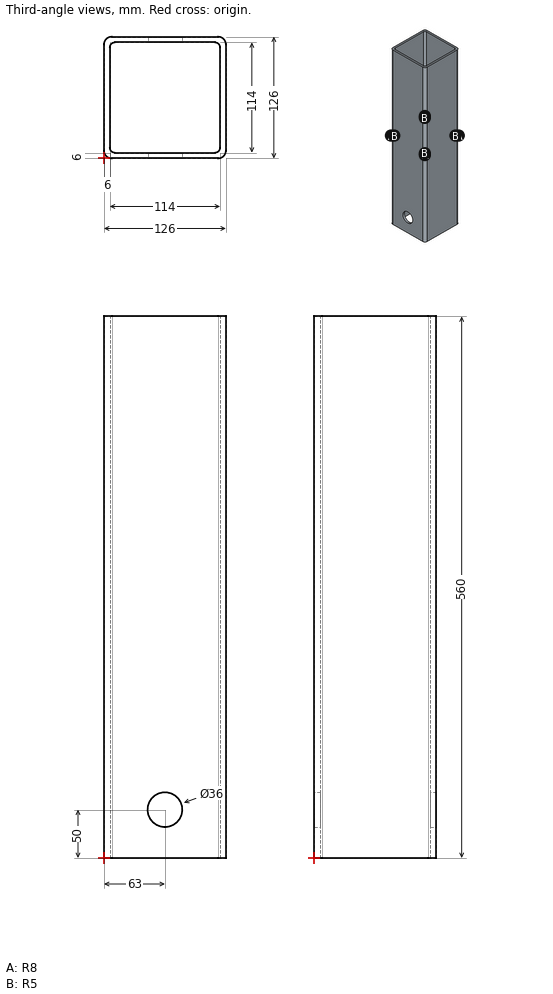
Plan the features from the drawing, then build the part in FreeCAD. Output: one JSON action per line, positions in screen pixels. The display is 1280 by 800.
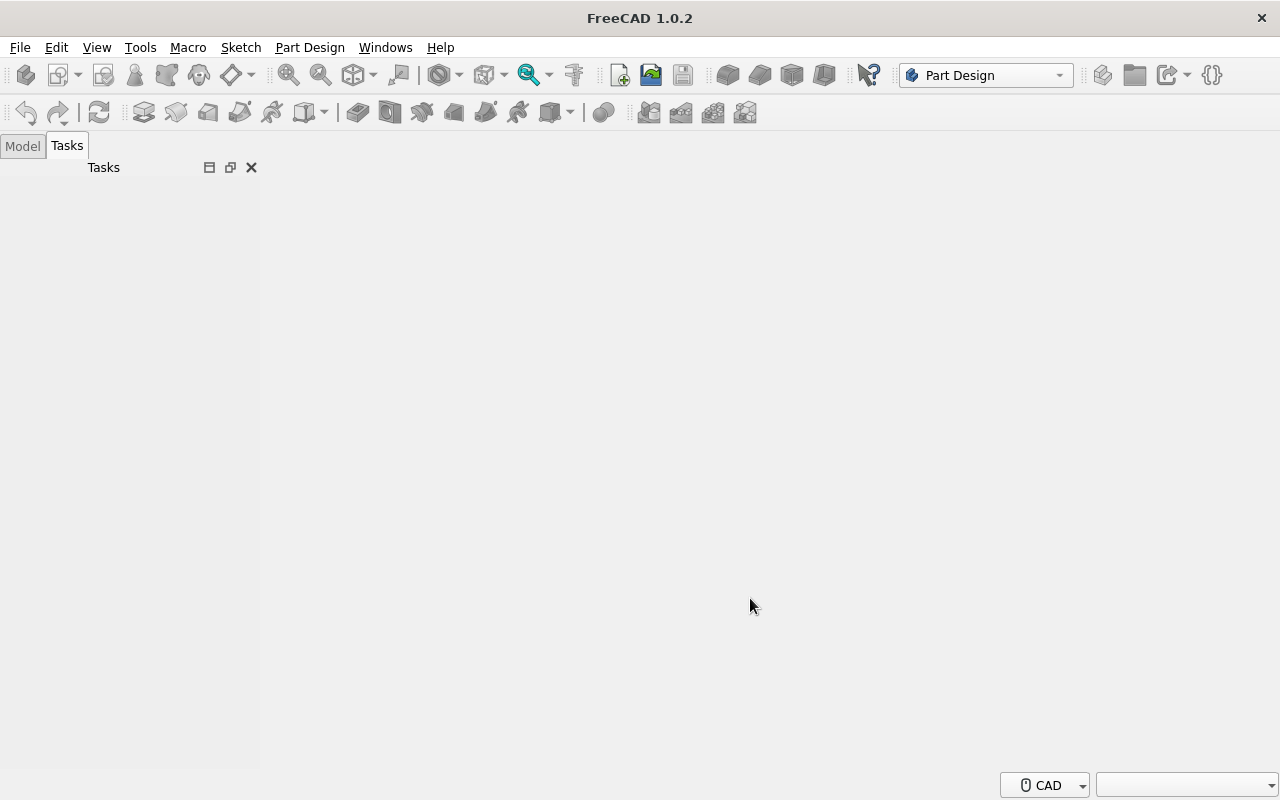
{"action": "left_click", "coordinate": [620, 76]}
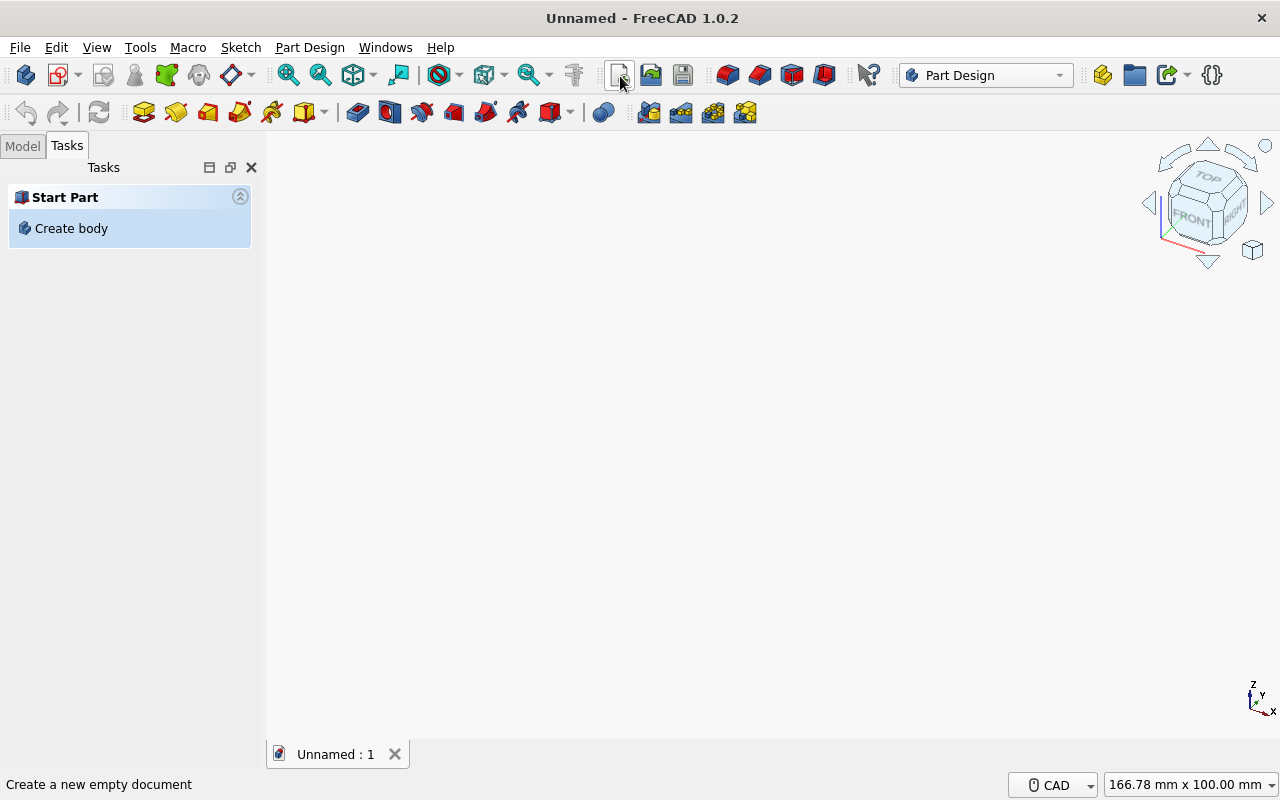
{"action": "left_click", "coordinate": [58, 76]}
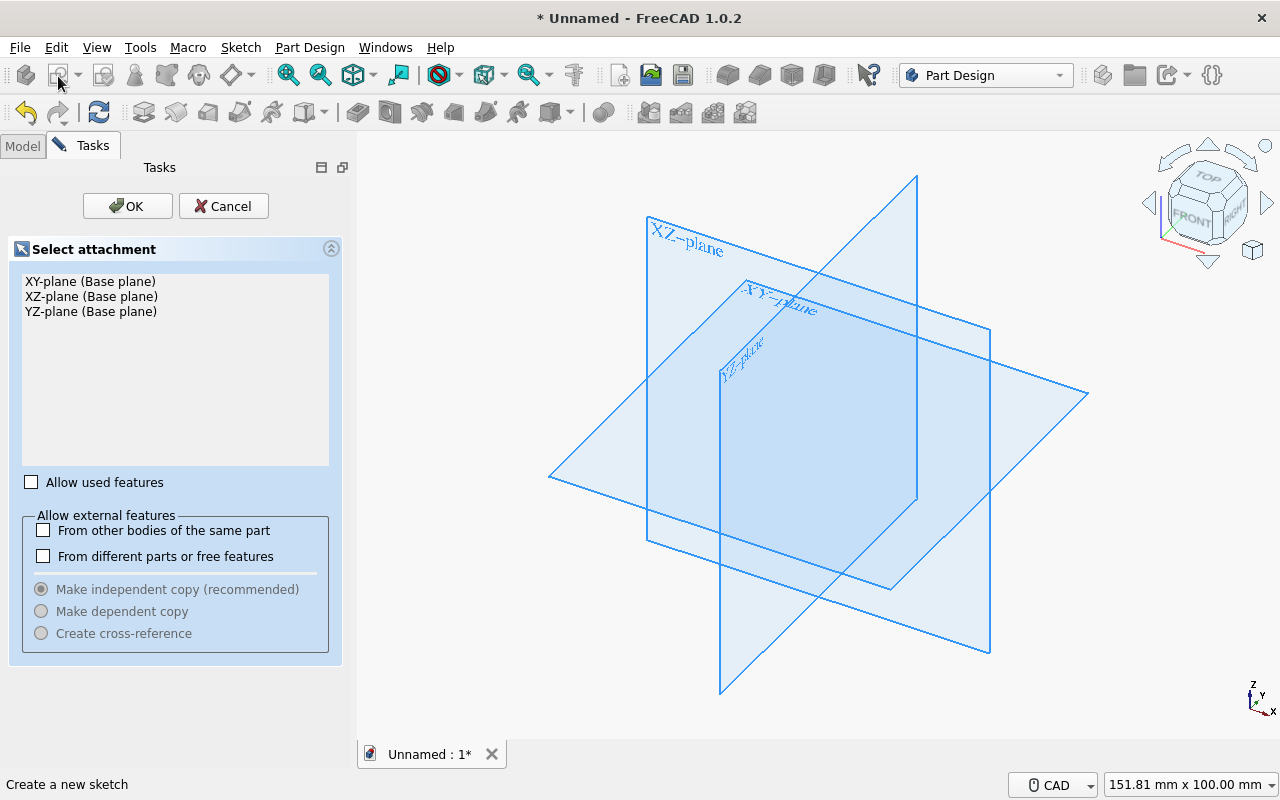
{"action": "left_click", "coordinate": [82, 282]}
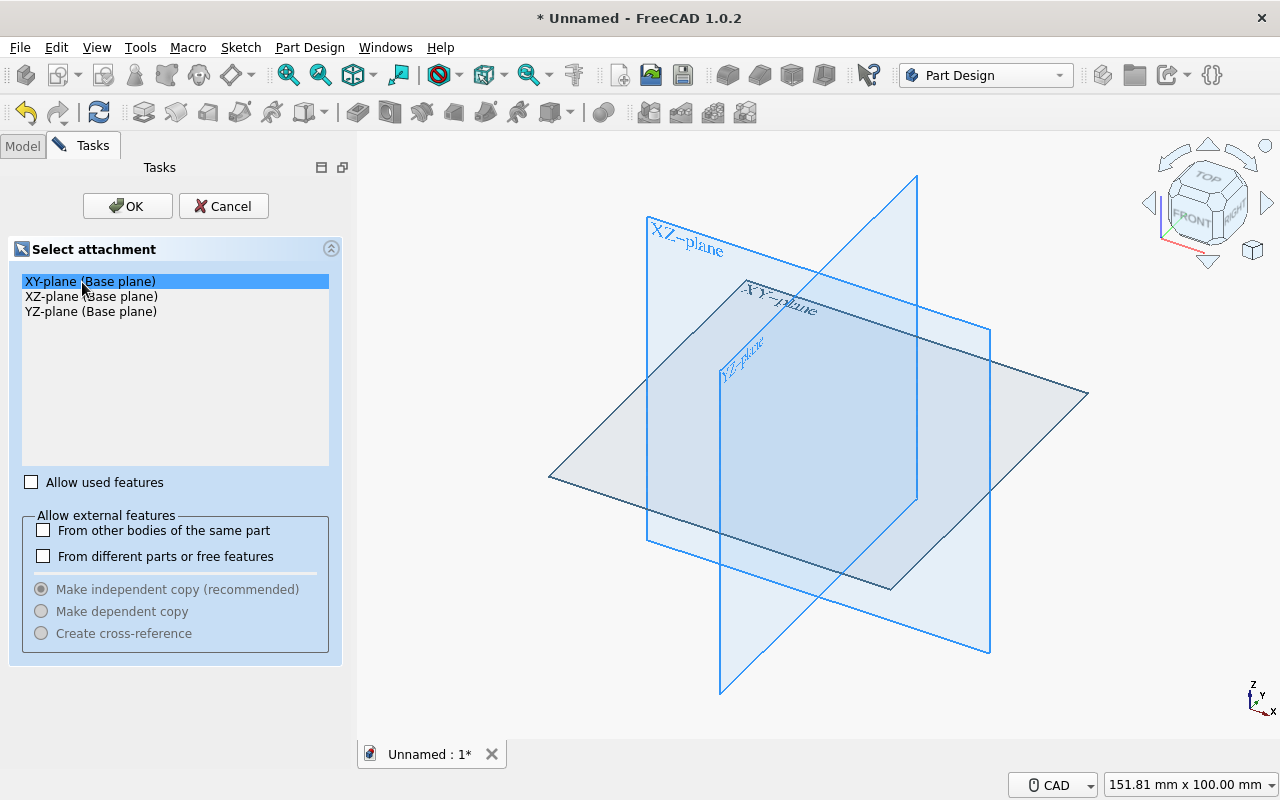
{"action": "left_click", "coordinate": [128, 206]}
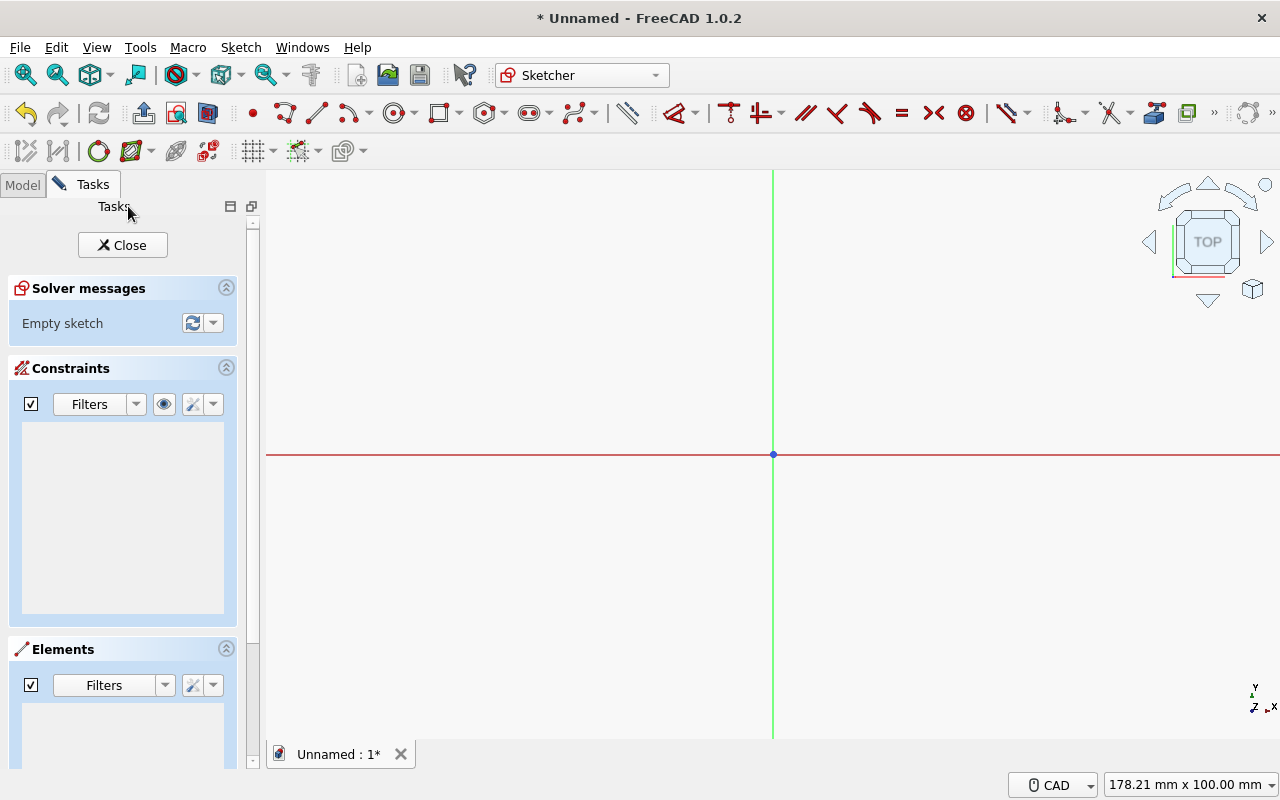
{"action": "scroll", "coordinate": [356, 711], "scroll_direction": "down", "scroll_amount": 4}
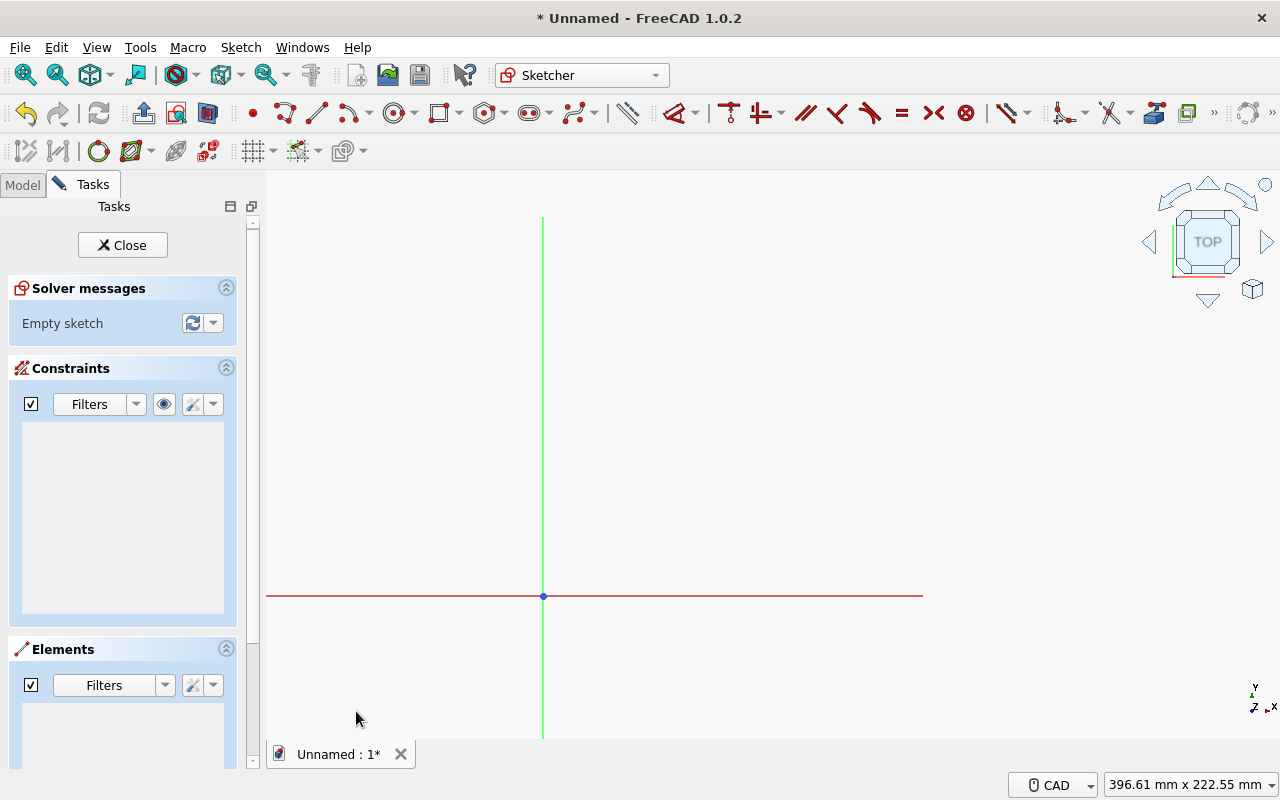
{"action": "left_click", "coordinate": [440, 114]}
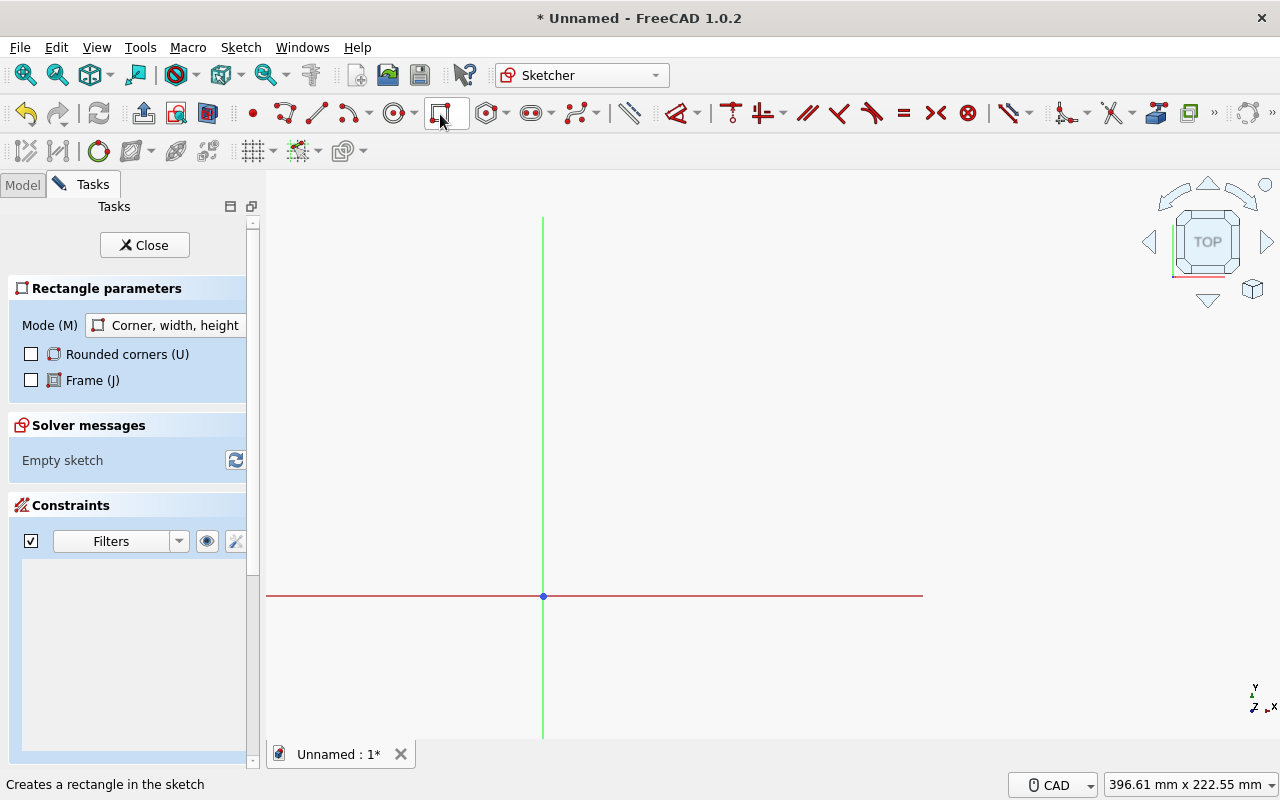
{"action": "left_click", "coordinate": [543, 596]}
{"action": "mouse_move", "coordinate": [866, 274]}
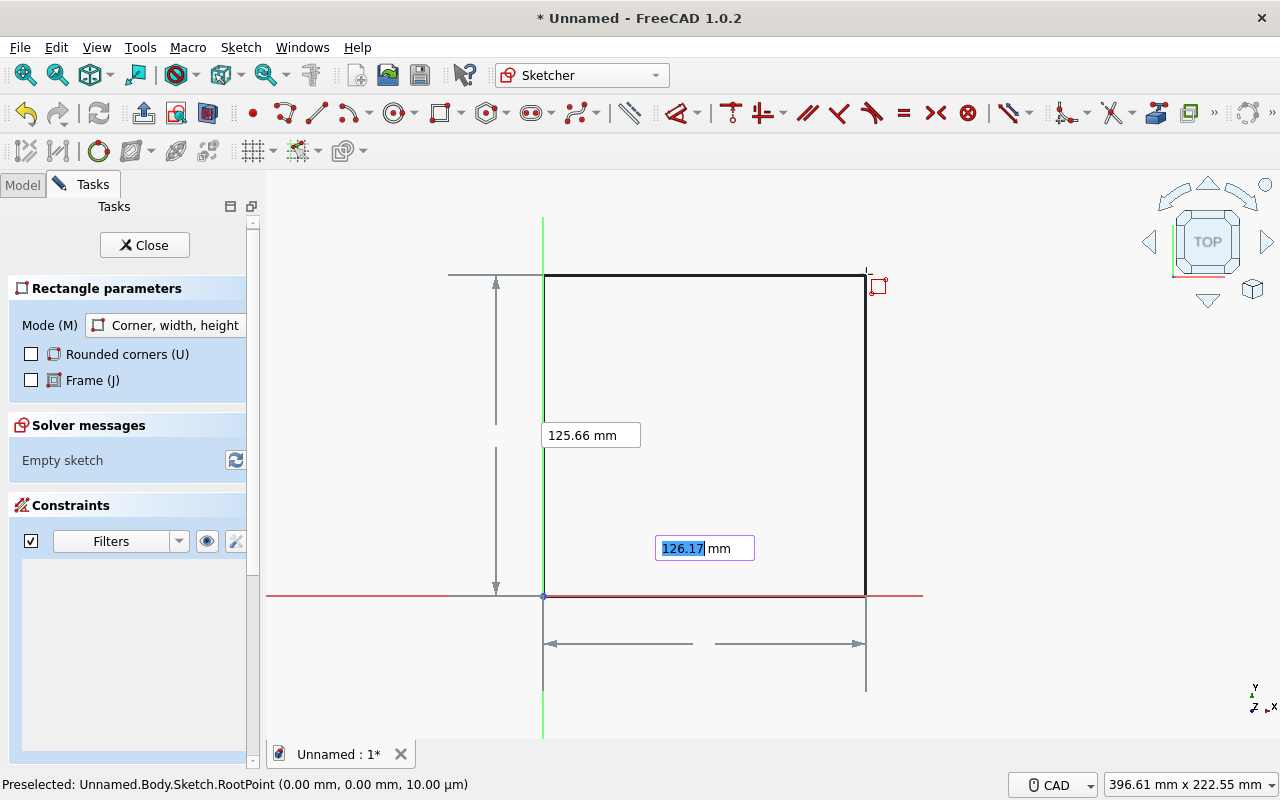
{"action": "type", "text": "126"}
{"action": "key", "text": "Tab"}
{"action": "type", "text": "126"}
{"action": "key", "text": "Return"}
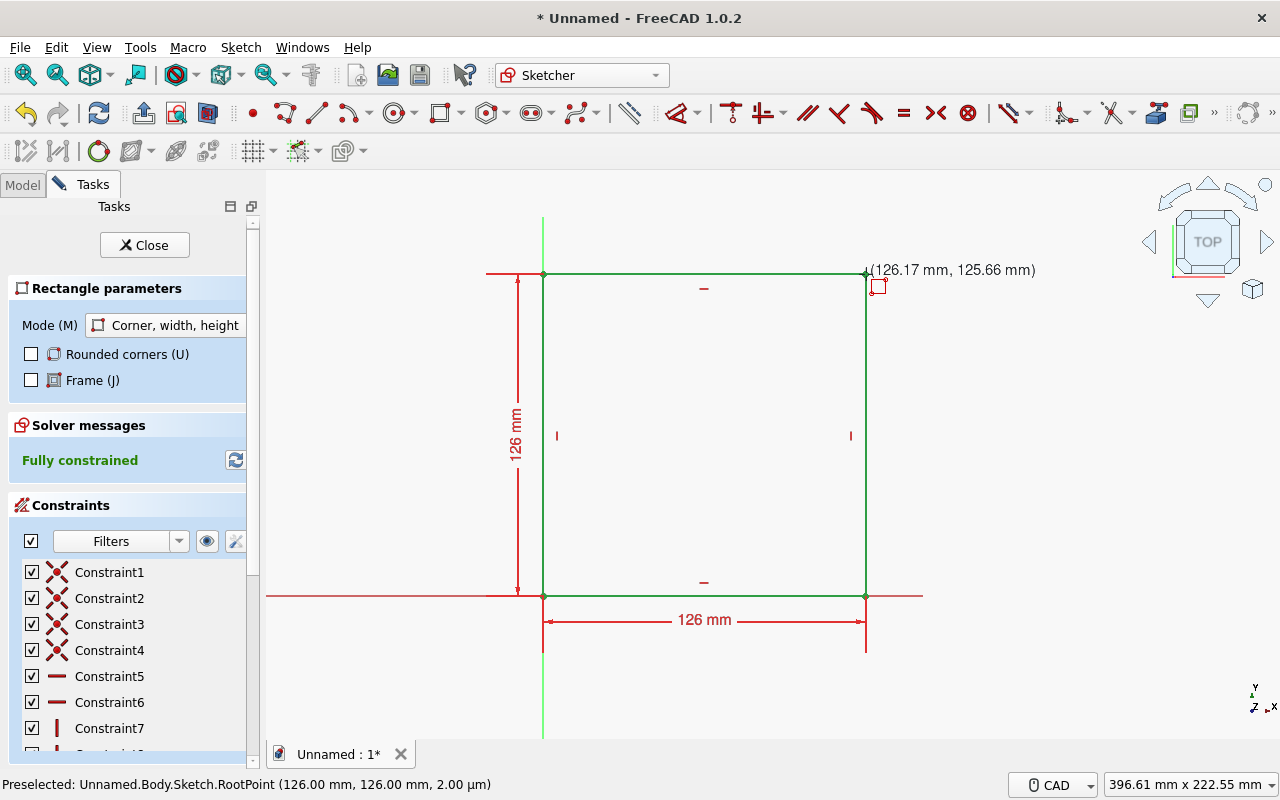
{"action": "left_click", "coordinate": [559, 289]}
{"action": "mouse_move", "coordinate": [850, 581]}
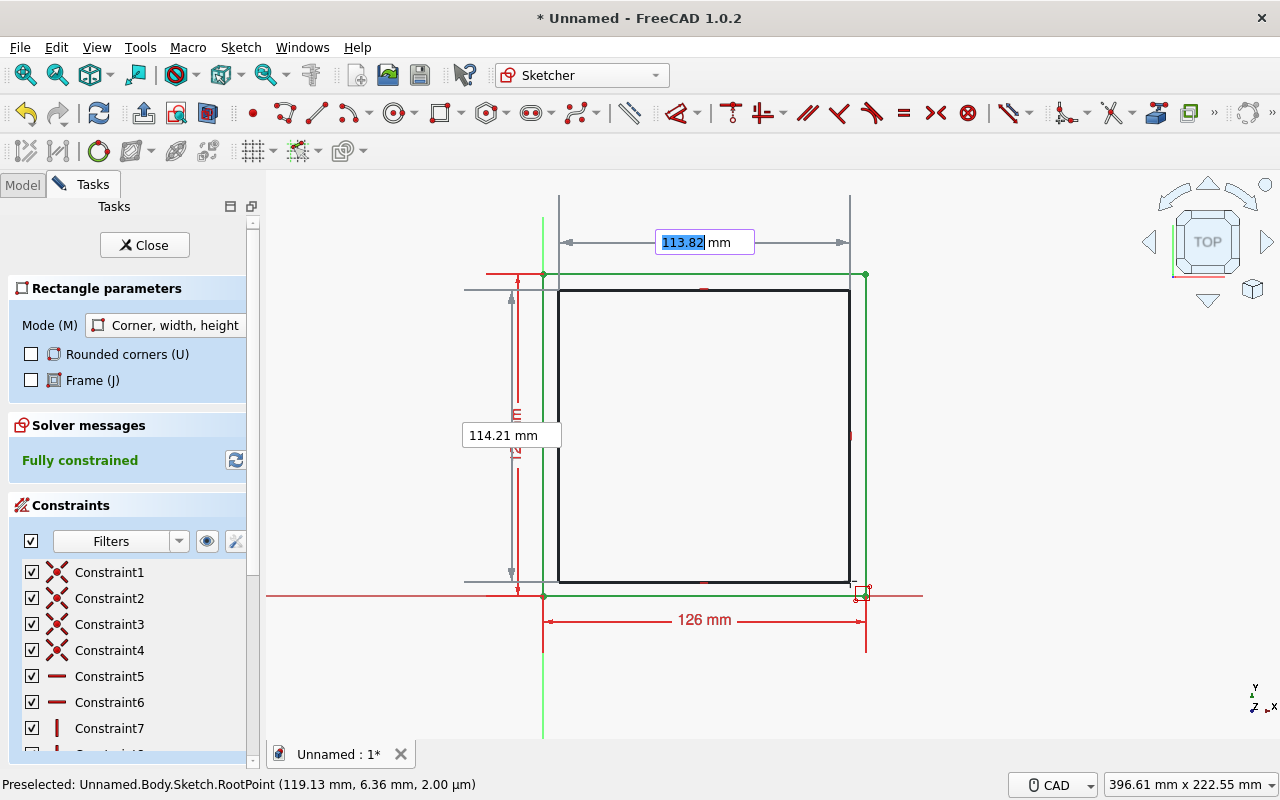
{"action": "type", "text": "114"}
{"action": "key", "text": "Tab"}
{"action": "type", "text": "114"}
{"action": "key", "text": "Return"}
{"action": "key", "text": "Escape"}